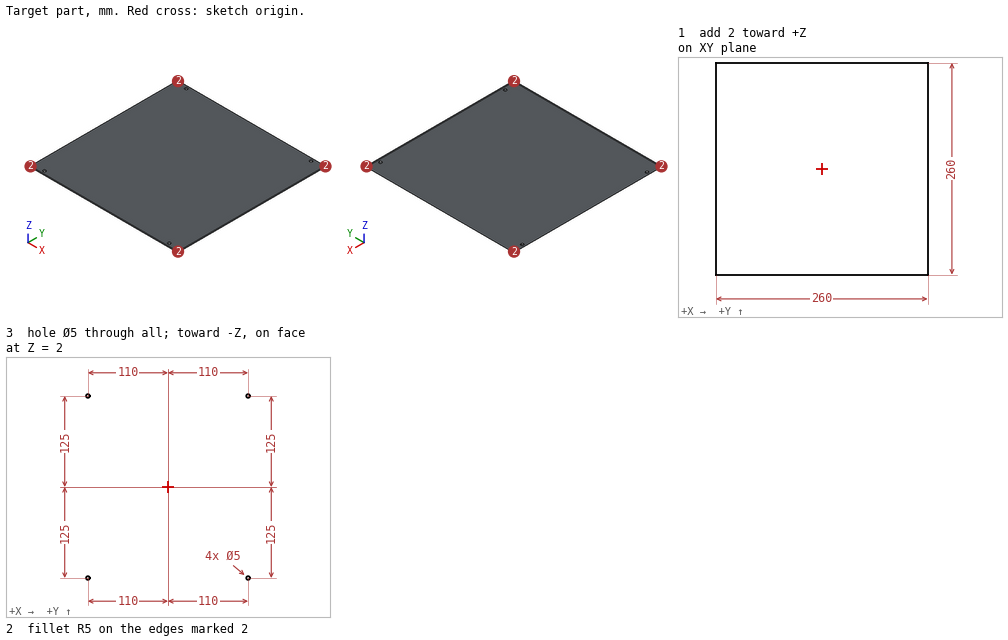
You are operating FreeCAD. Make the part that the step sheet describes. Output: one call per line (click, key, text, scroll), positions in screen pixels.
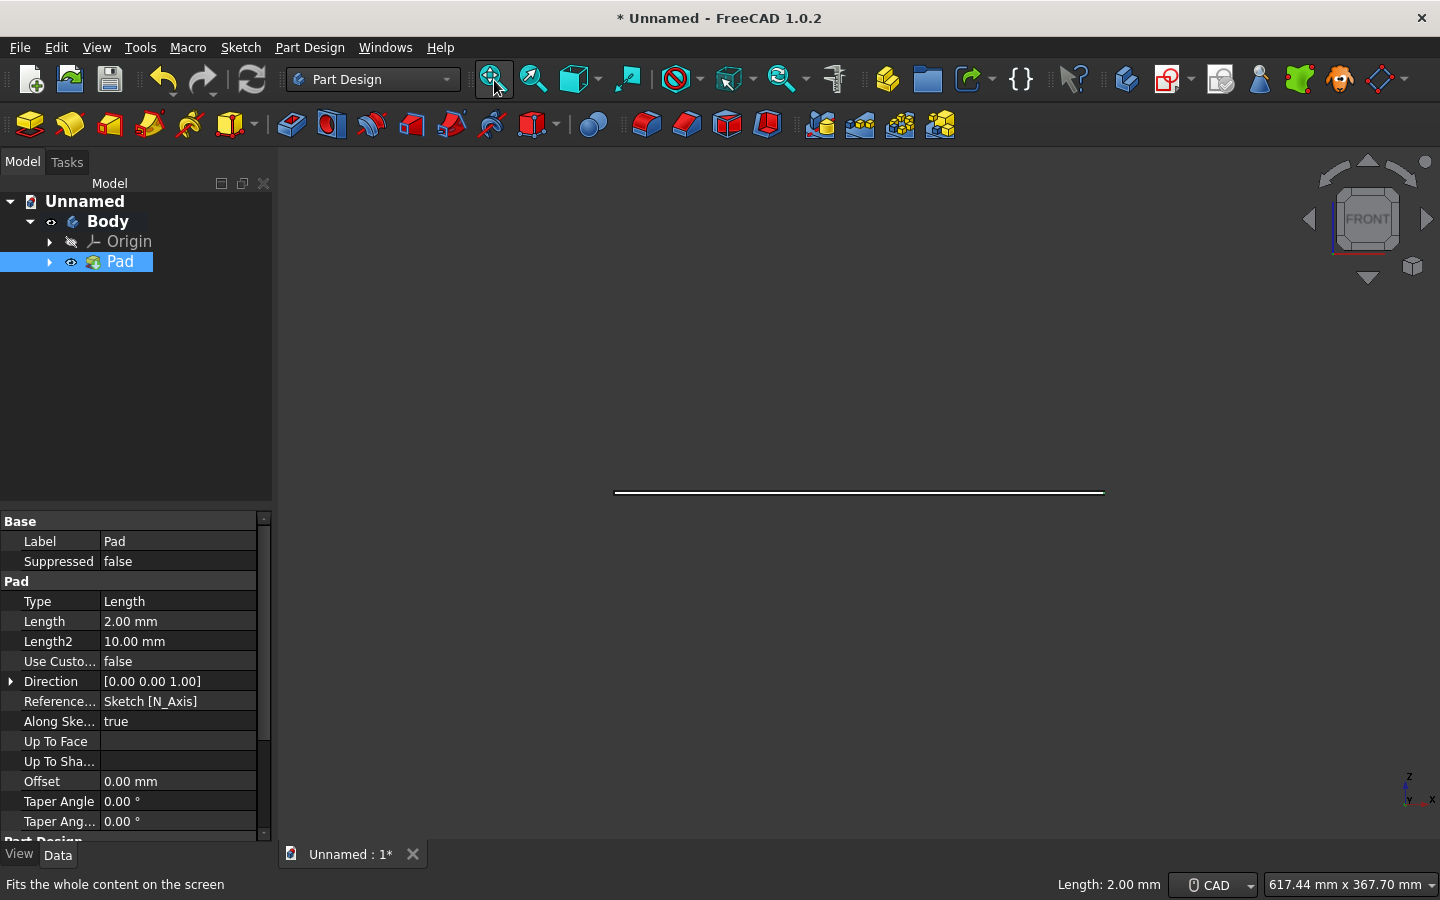
click(494, 80)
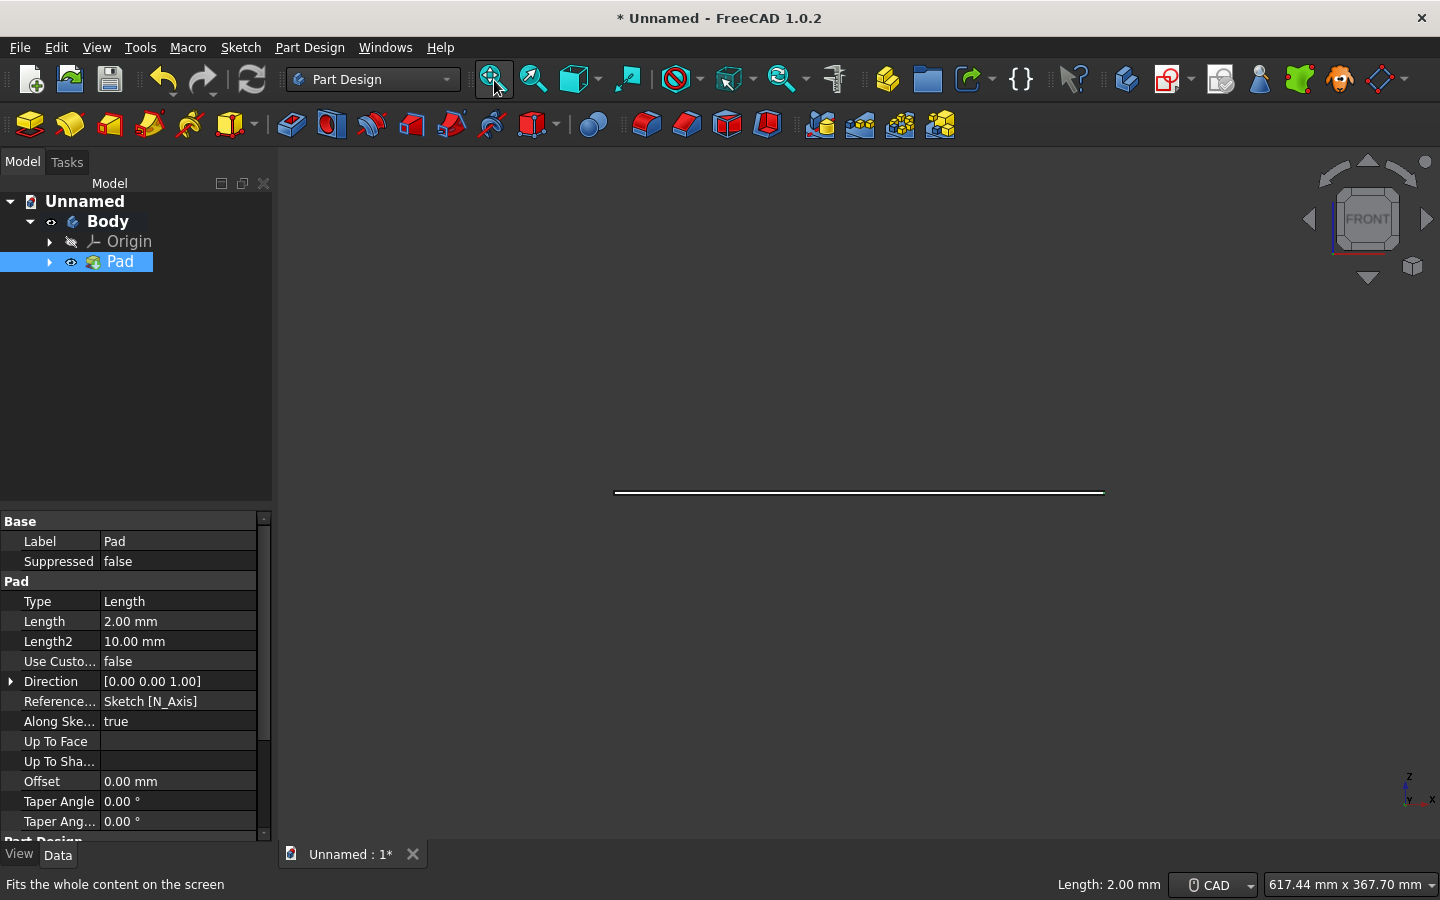
scroll(614, 492, up, 12)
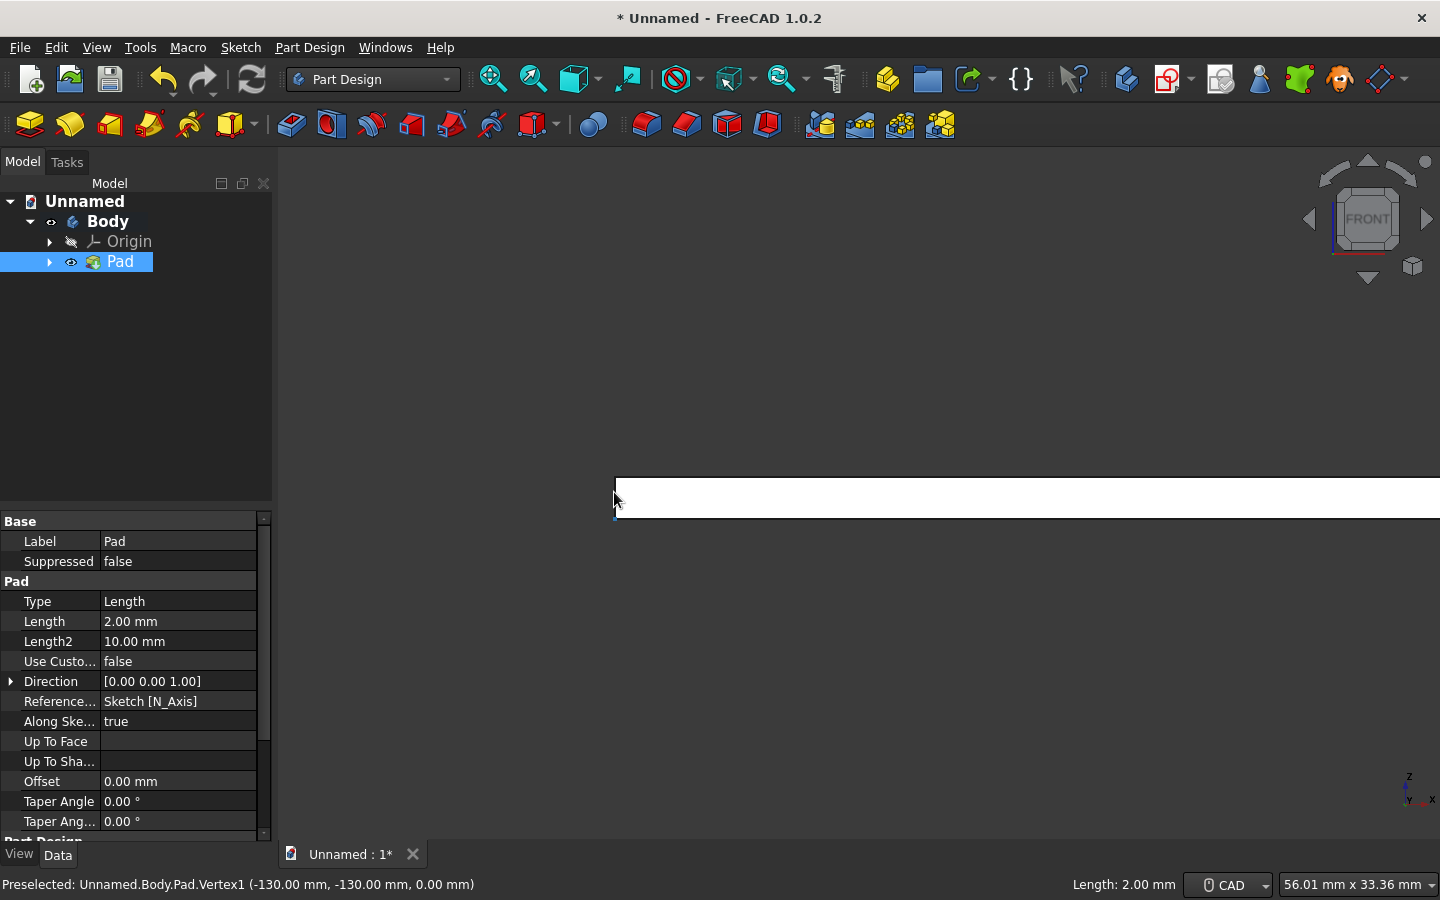
click(615, 497, ctrl)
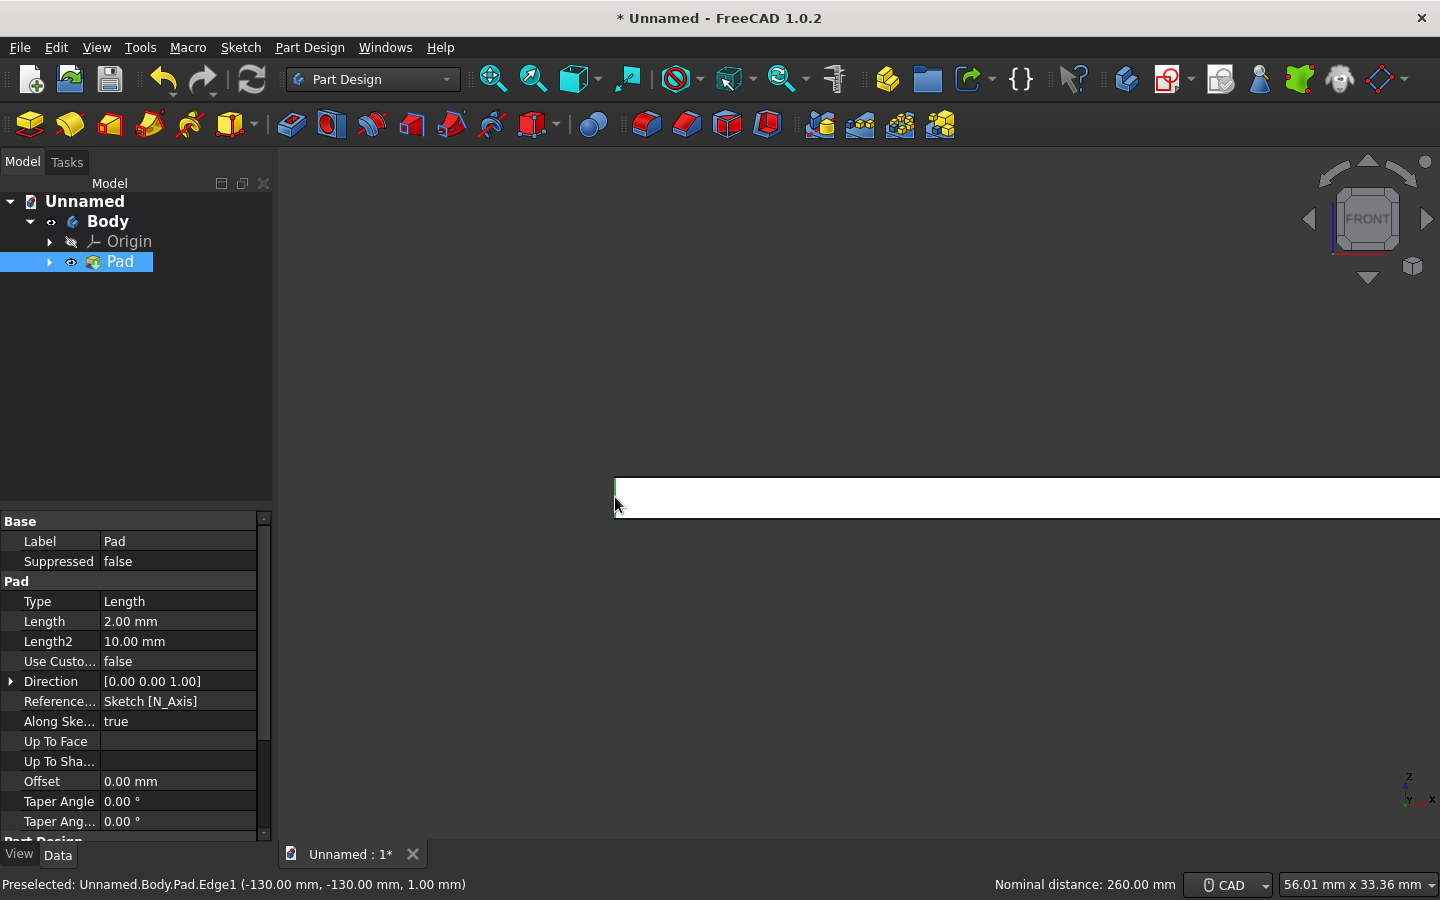
click(494, 80)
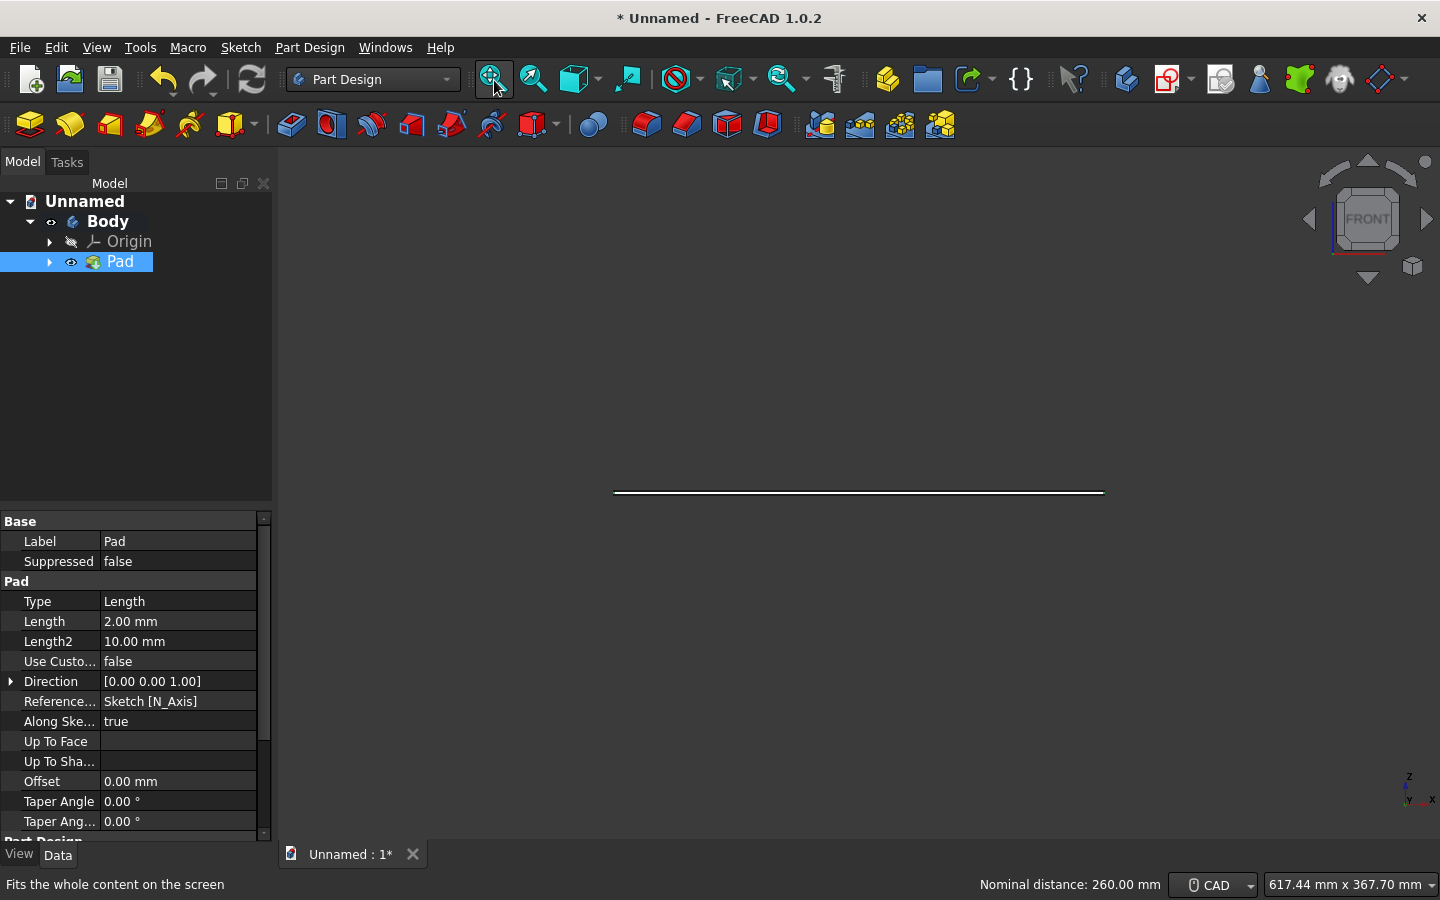
key(3)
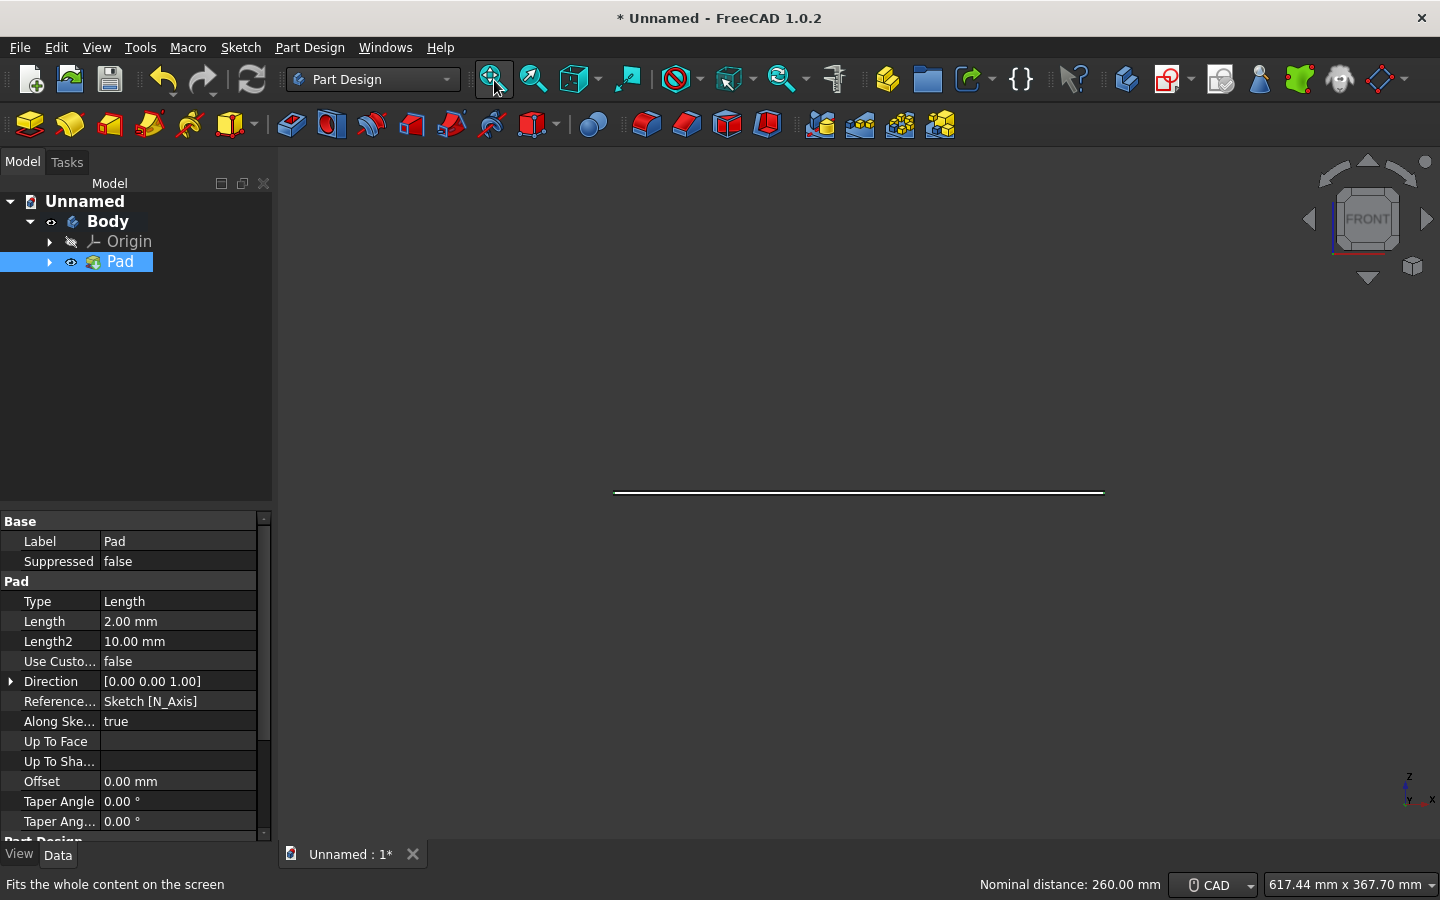
click(494, 80)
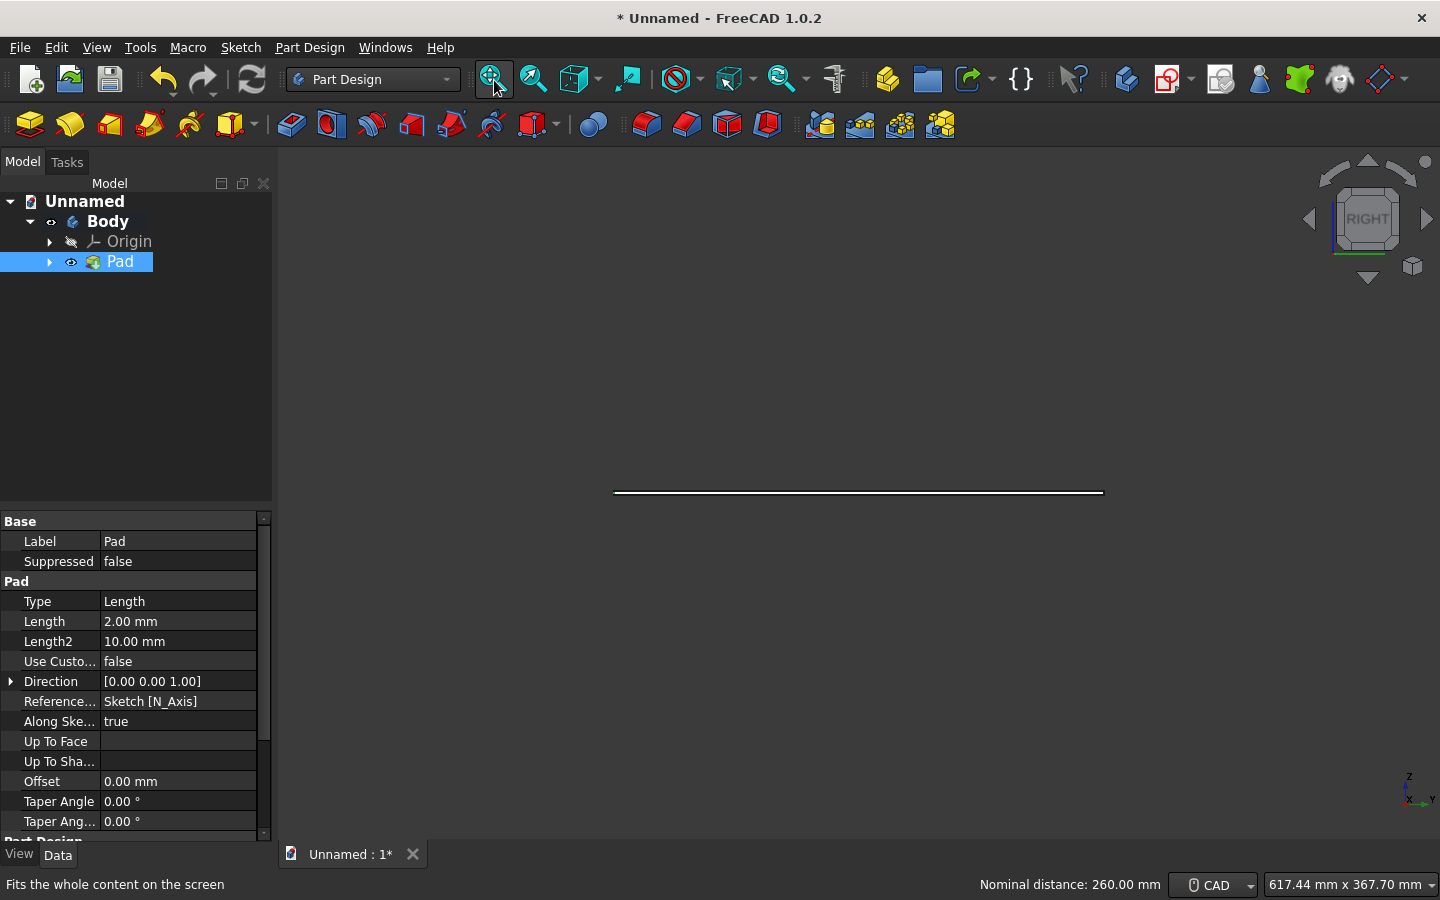
scroll(1104, 492, up, 12)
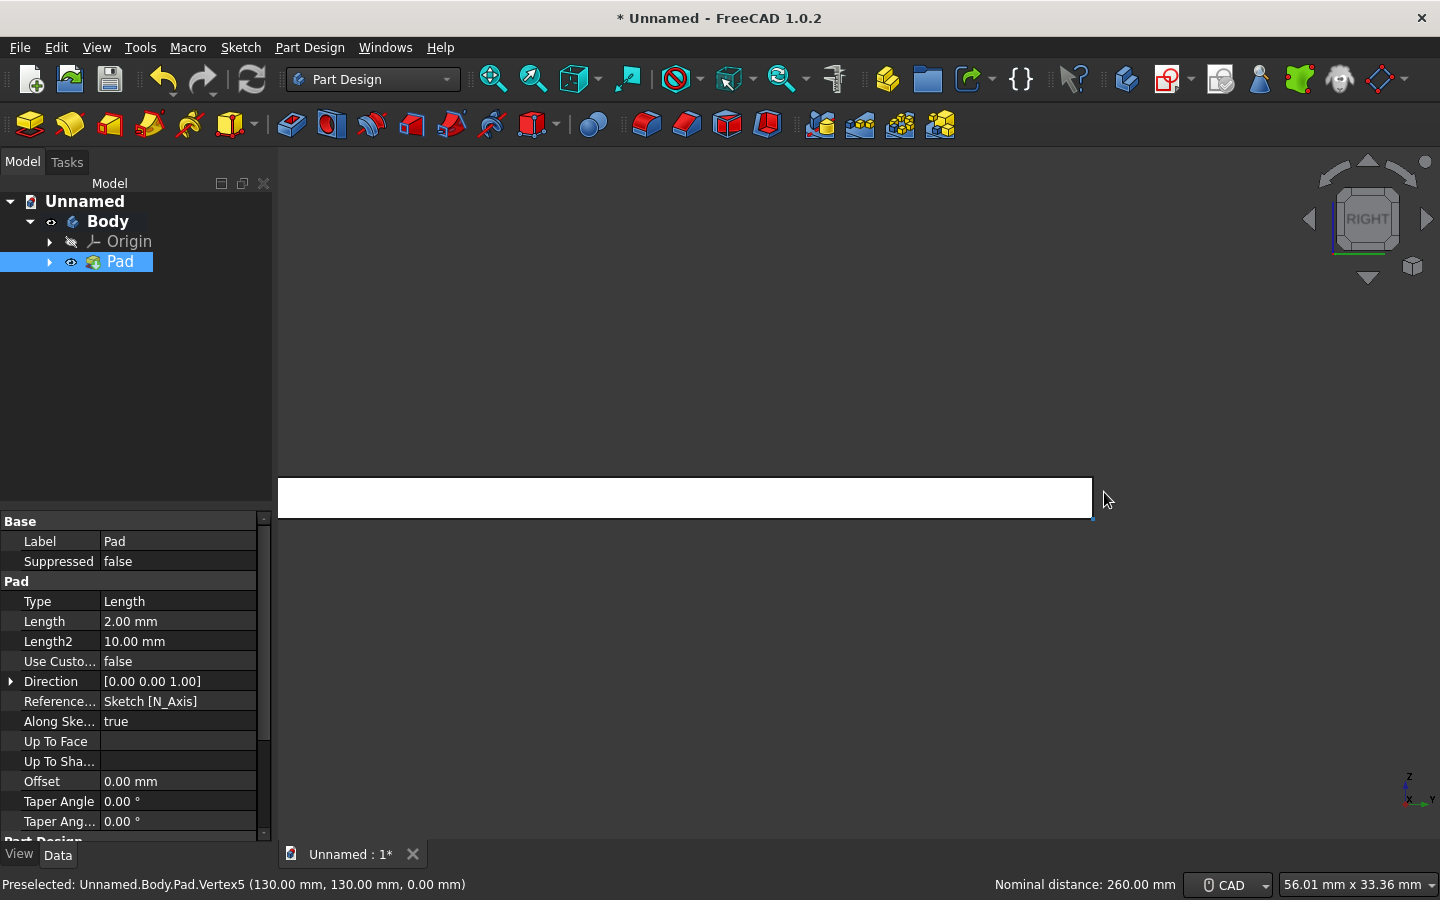
click(1093, 497, ctrl)